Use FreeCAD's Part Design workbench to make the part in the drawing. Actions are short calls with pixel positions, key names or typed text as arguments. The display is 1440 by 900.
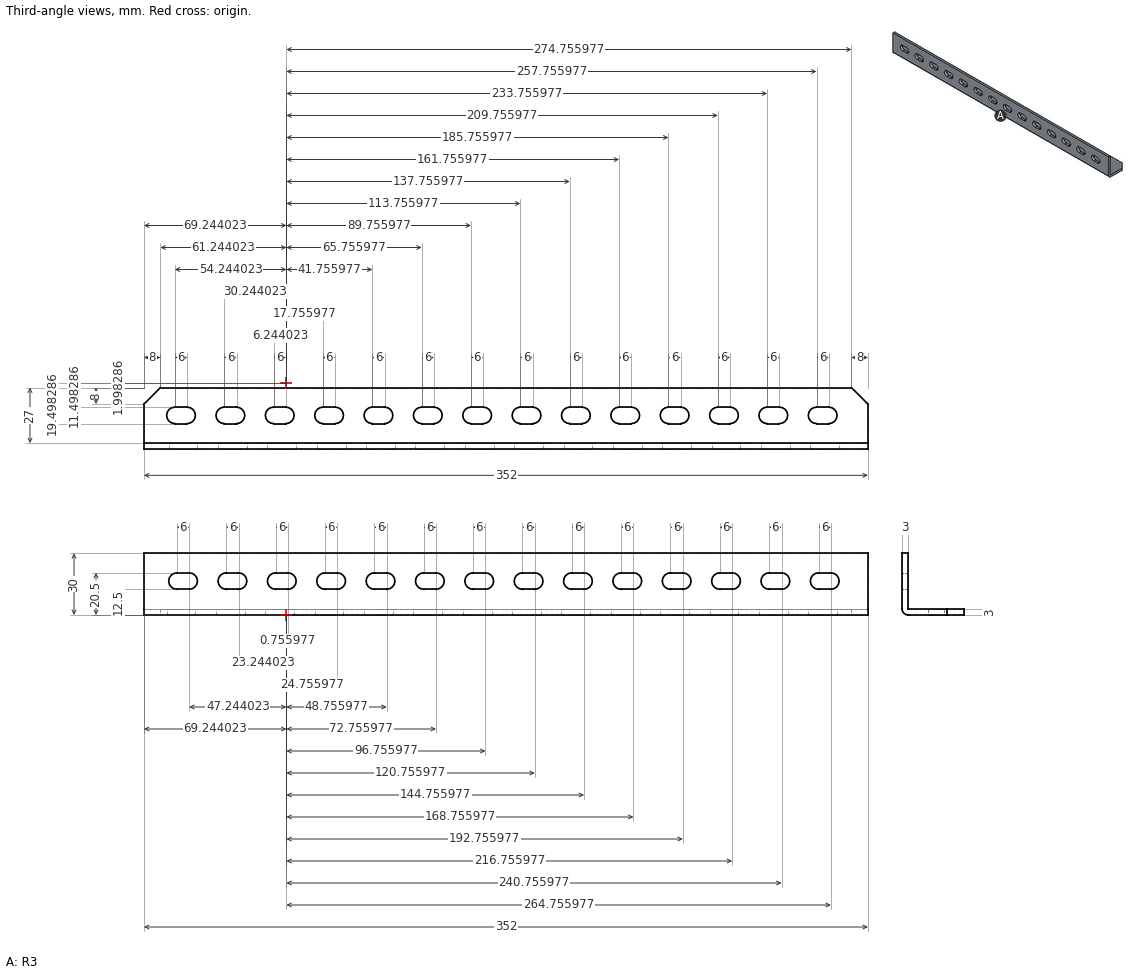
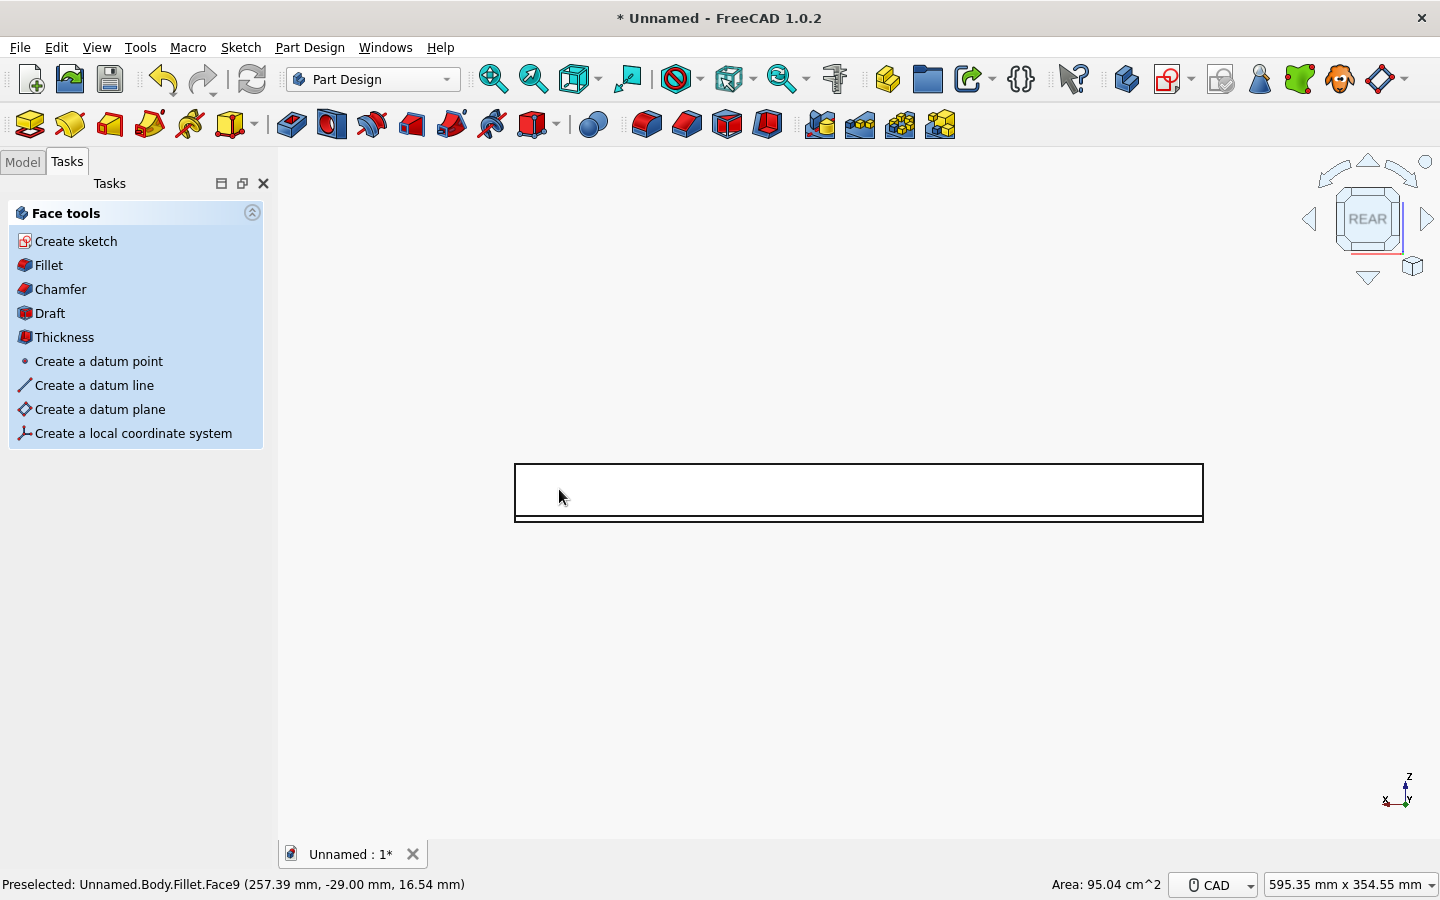
click(1168, 80)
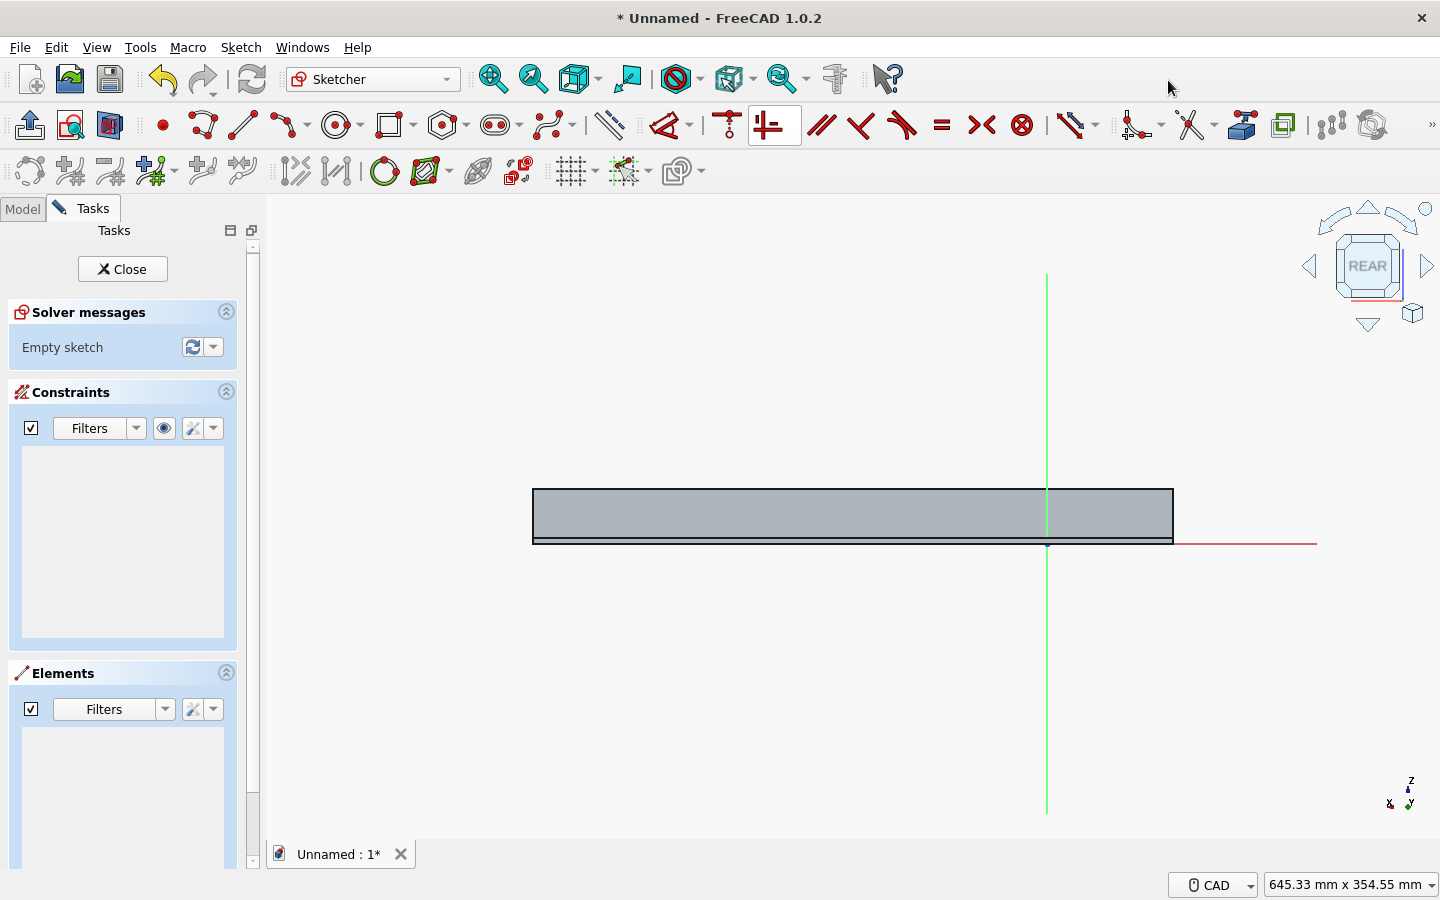
click(110, 126)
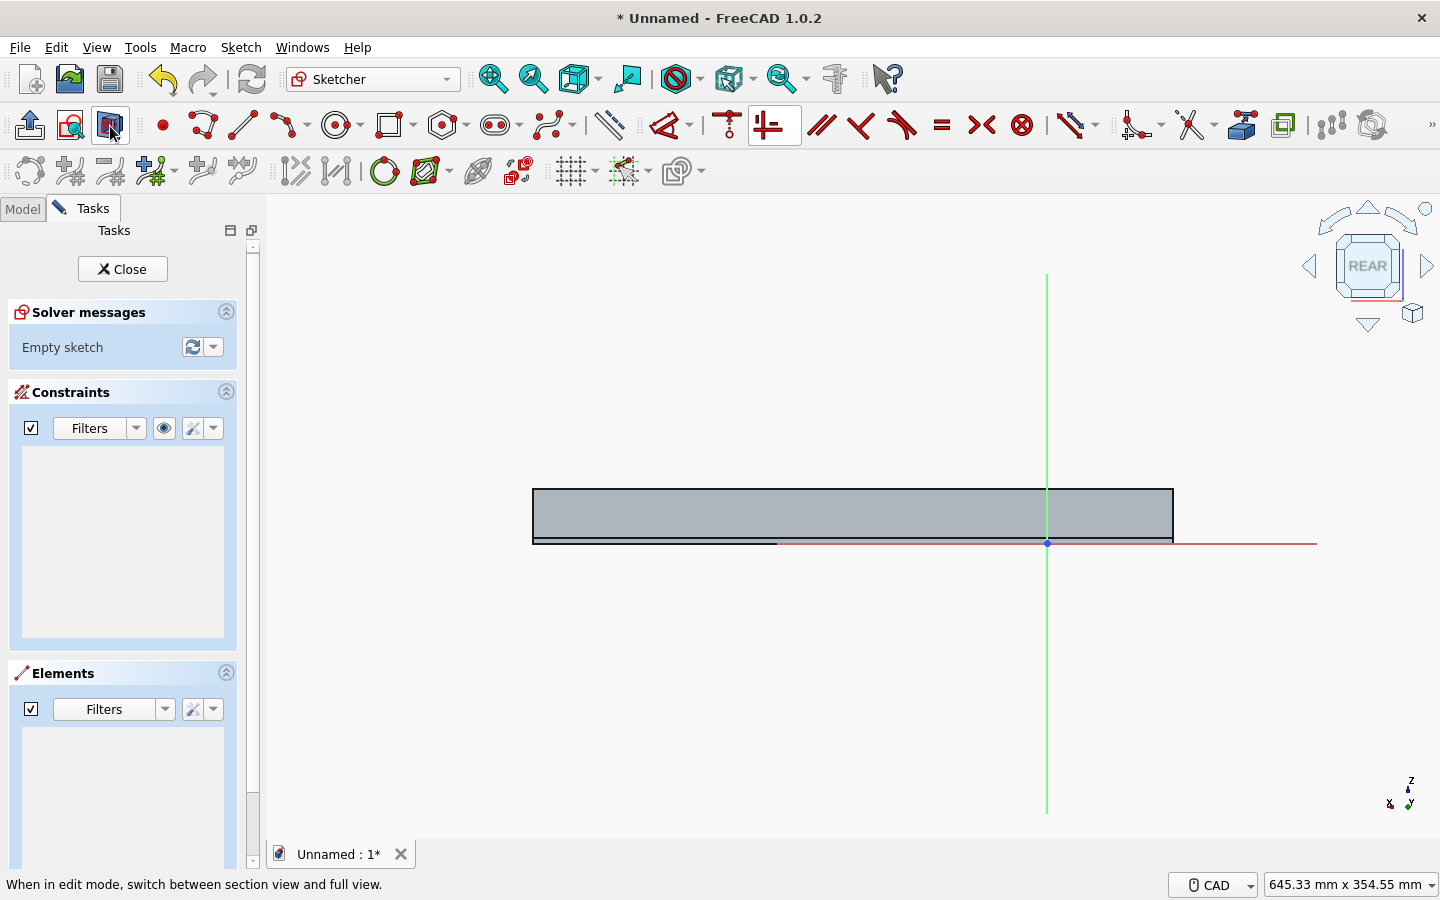
click(496, 126)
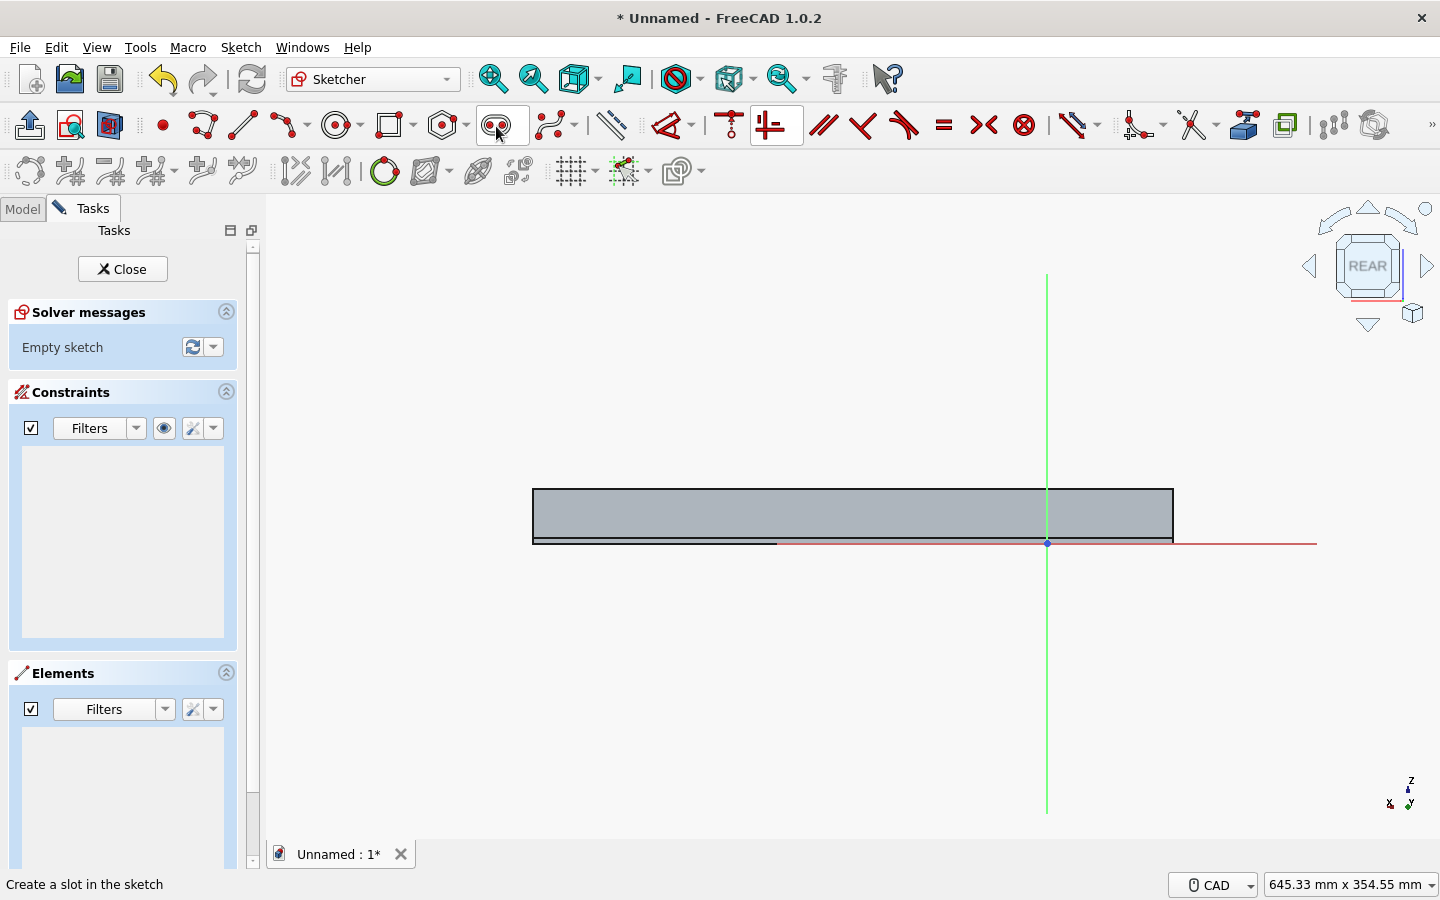
scroll(1133, 514, up, 6)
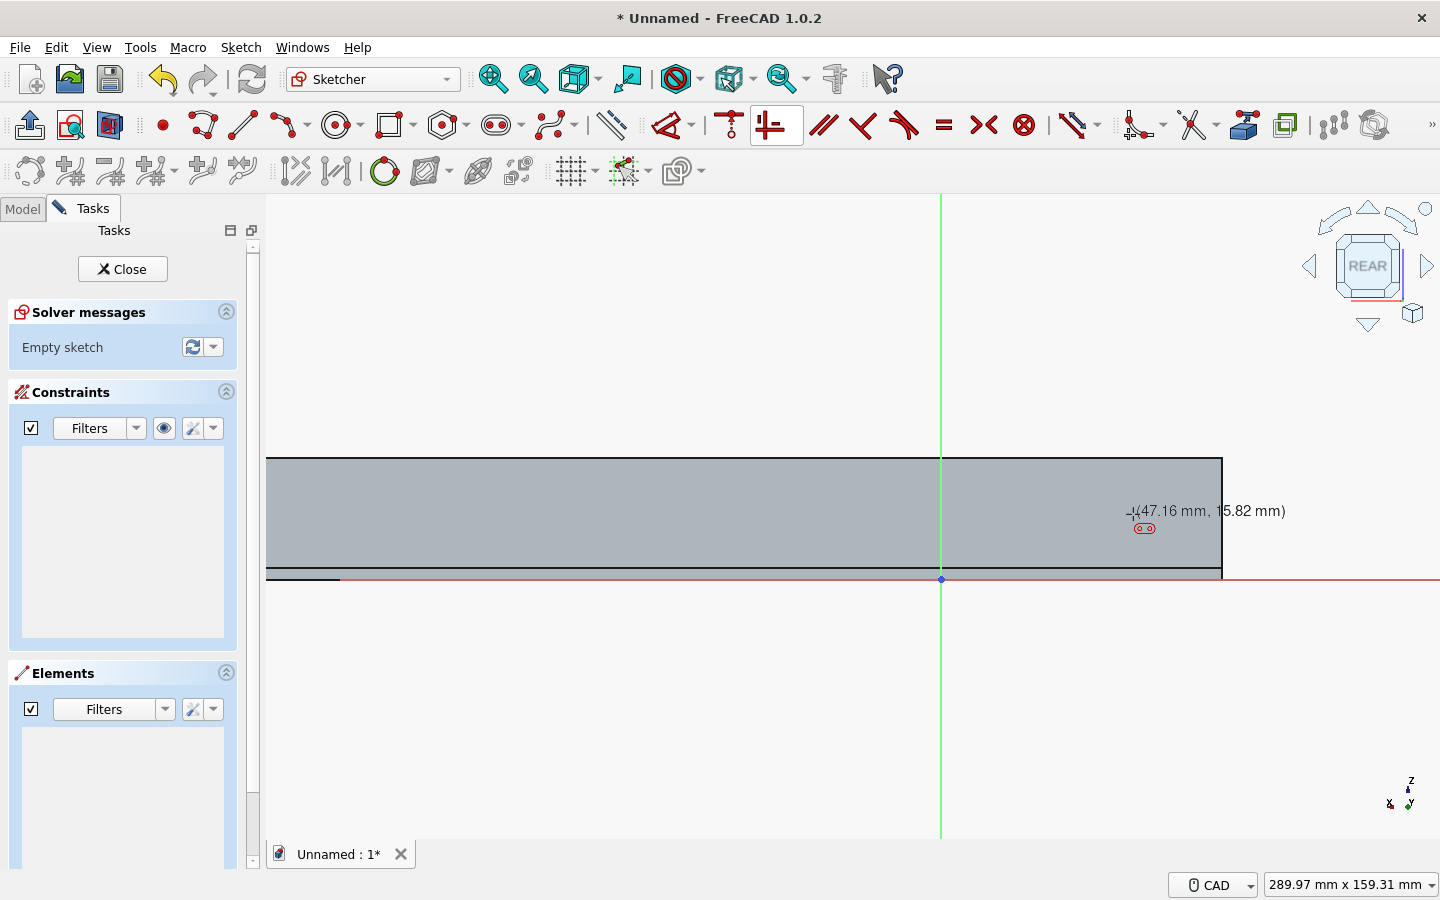
click(1132, 512)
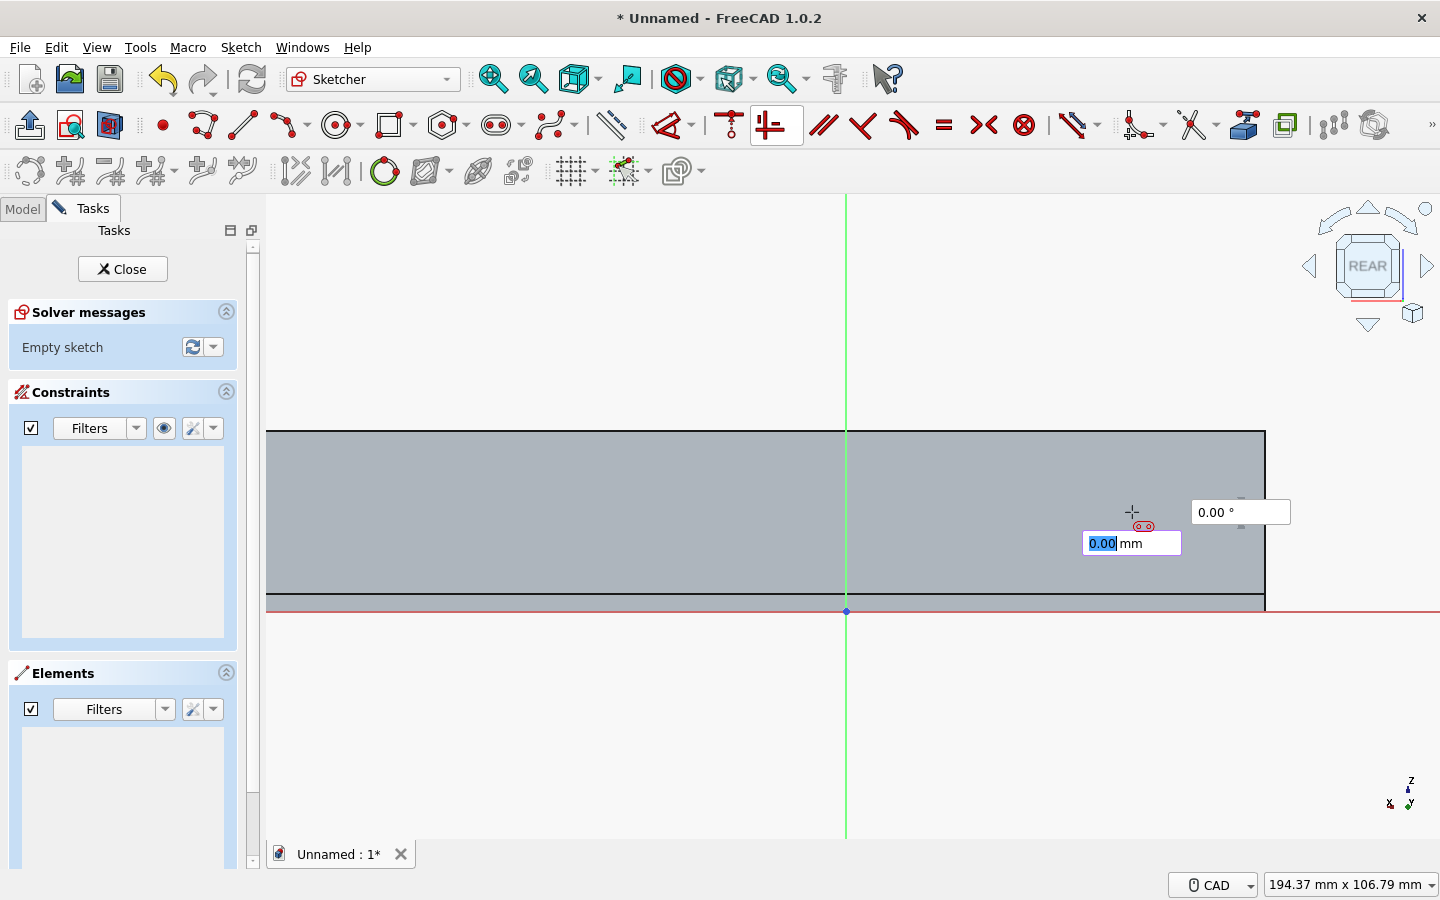
click(1168, 512)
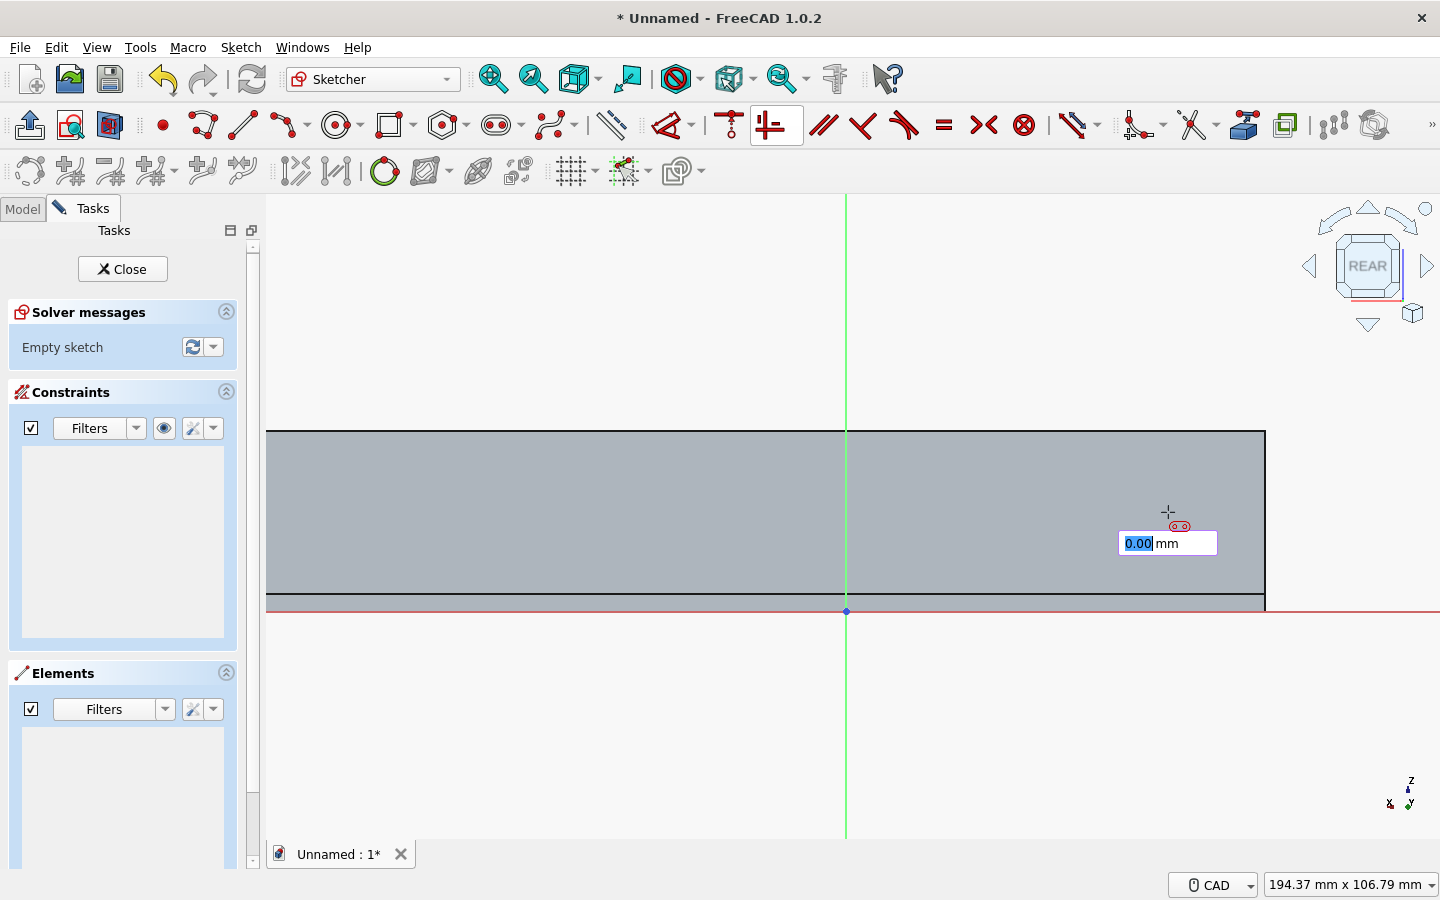
click(1150, 536)